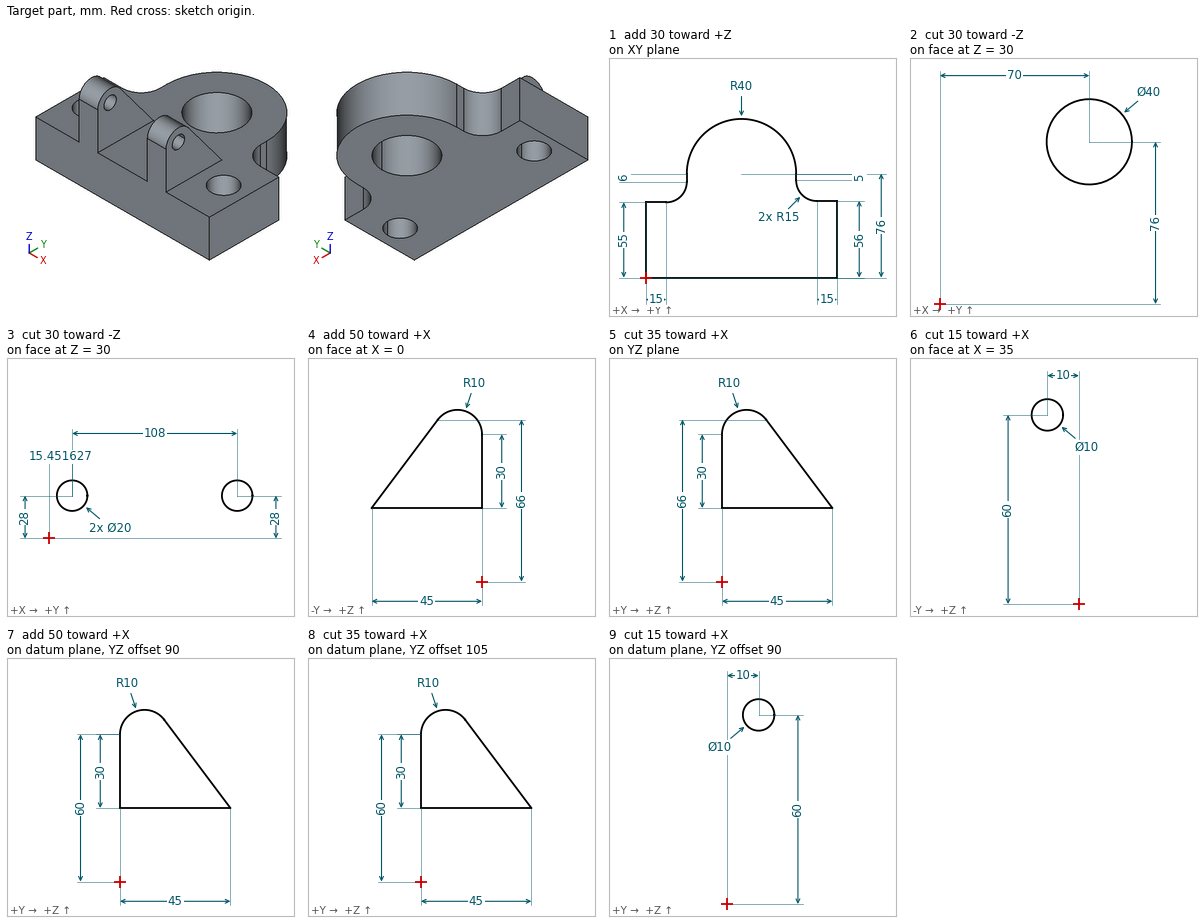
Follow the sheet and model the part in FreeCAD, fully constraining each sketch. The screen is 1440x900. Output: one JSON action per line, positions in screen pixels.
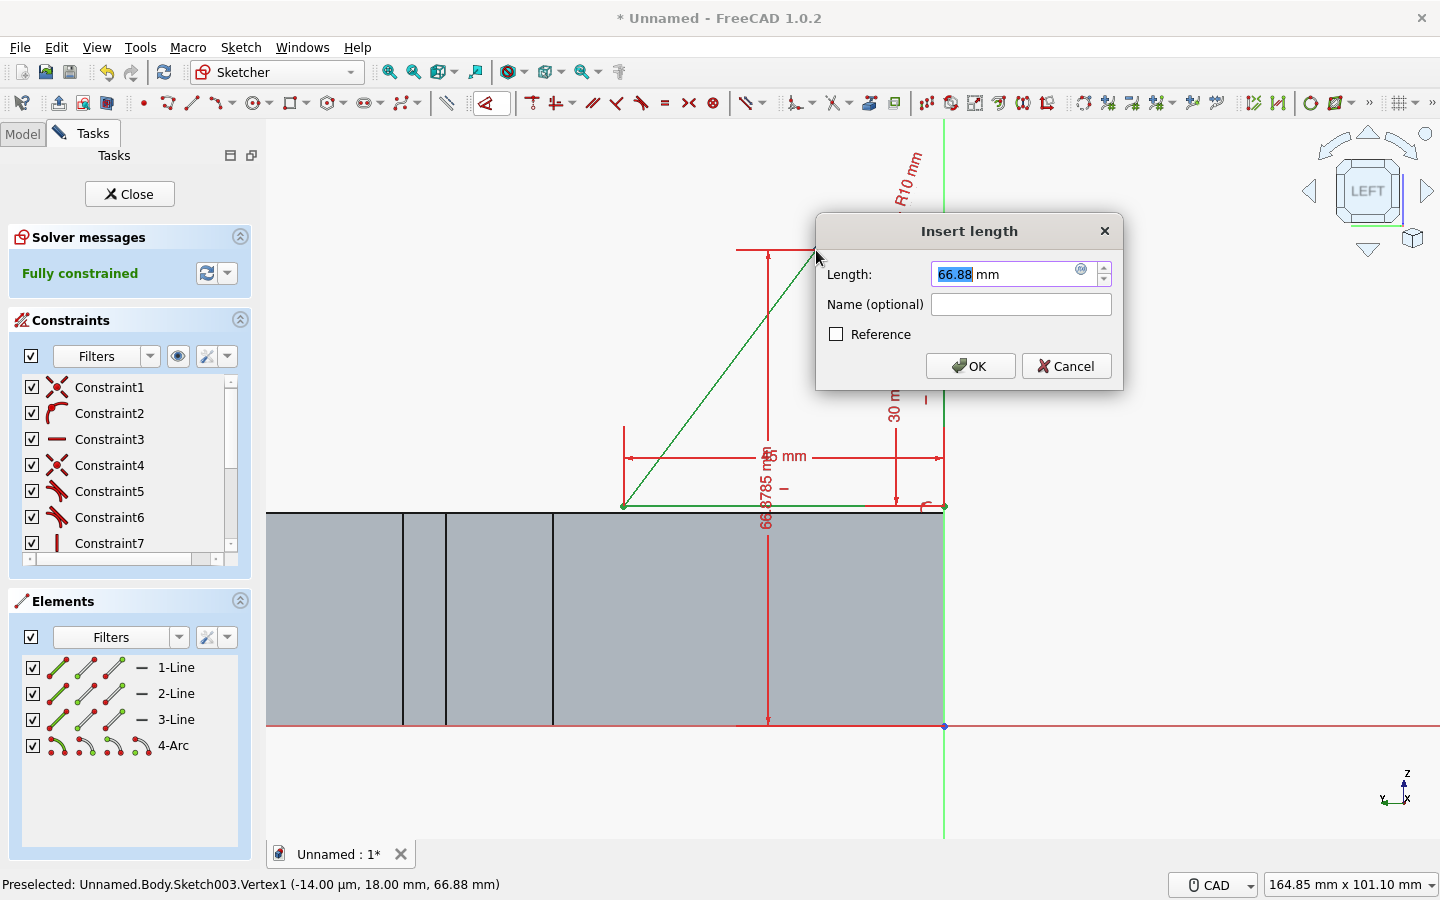
{"action": "type", "text": "66"}
{"action": "key", "text": "Return"}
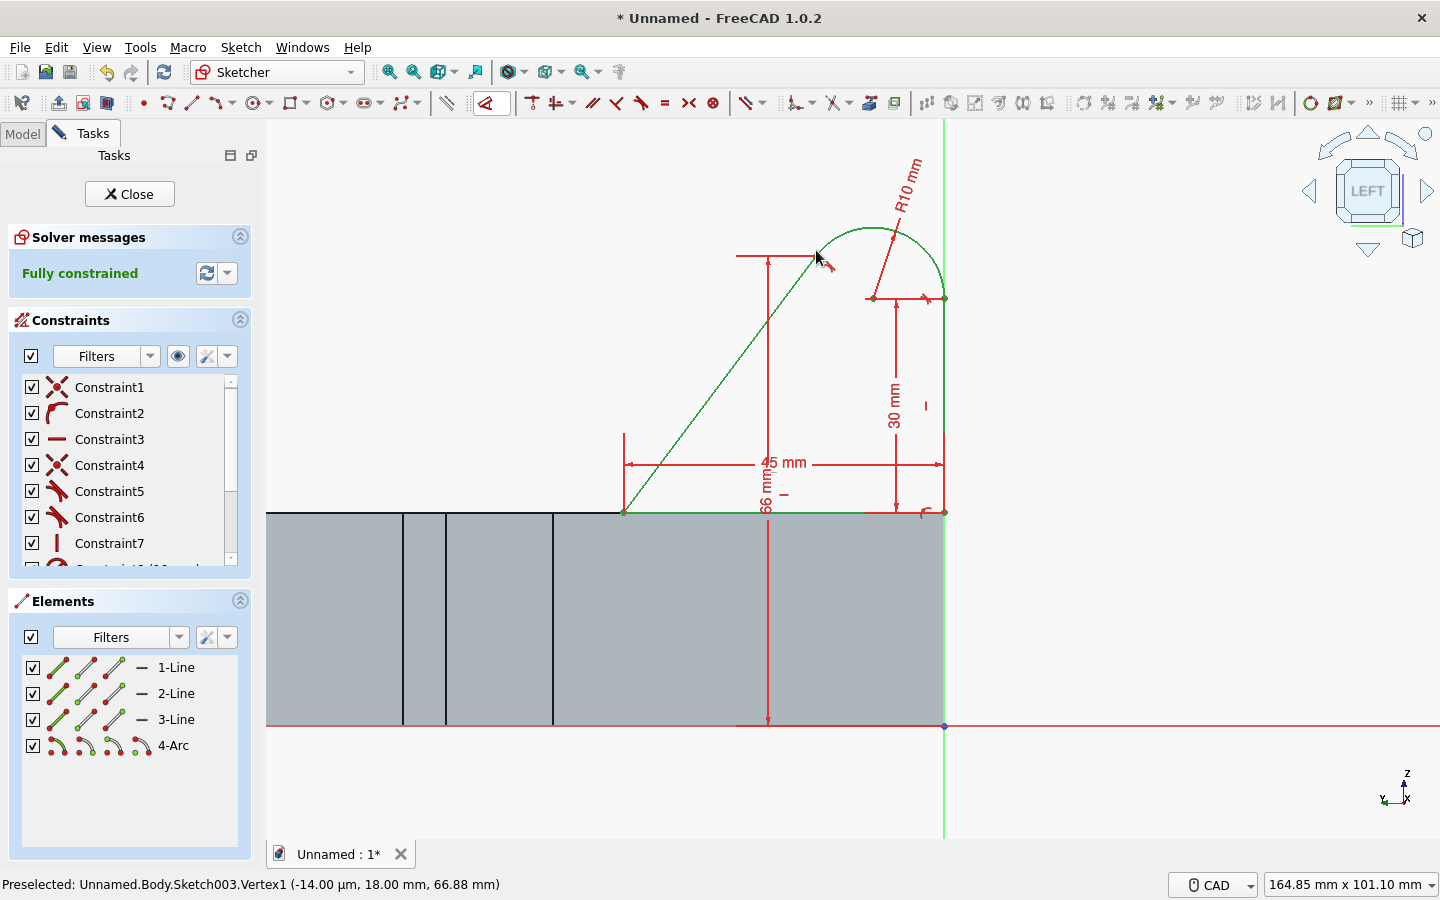
{"action": "left_click", "coordinate": [130, 194]}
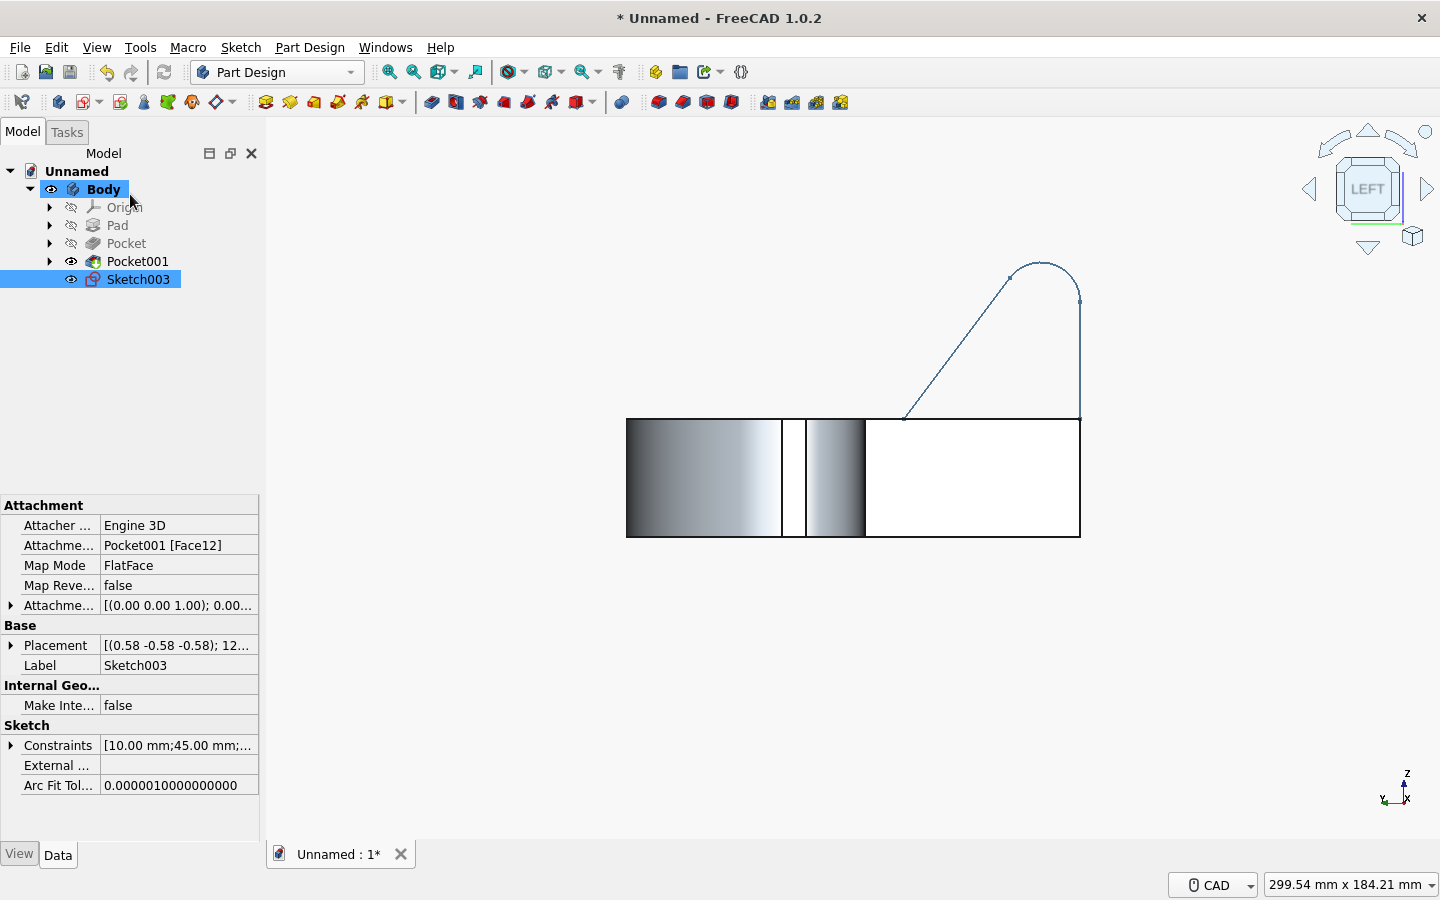
{"action": "left_click", "coordinate": [266, 102]}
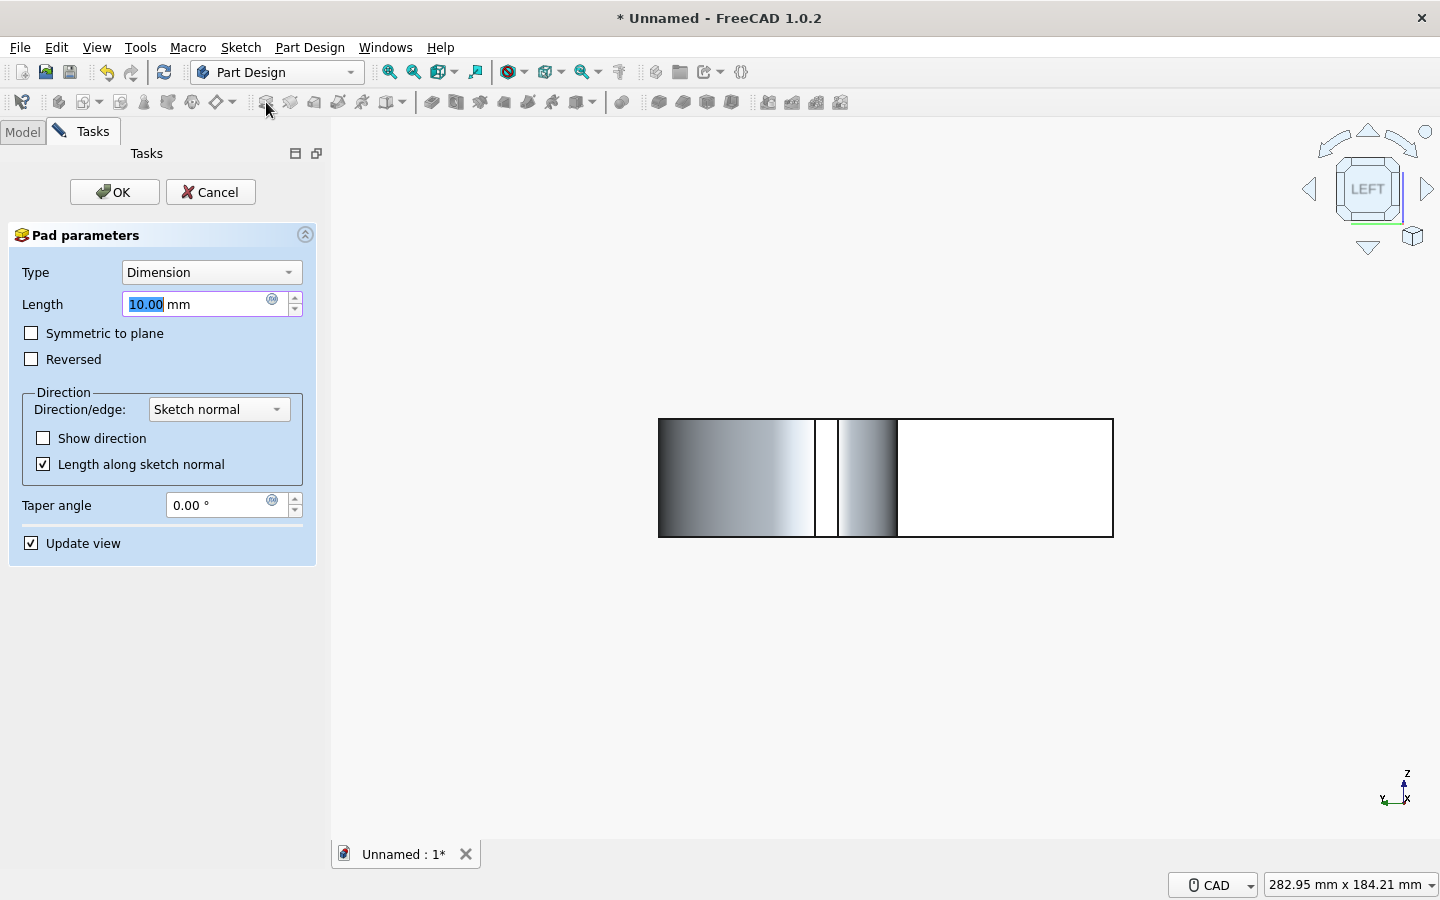
{"action": "type", "text": "50"}
{"action": "key", "text": "Tab"}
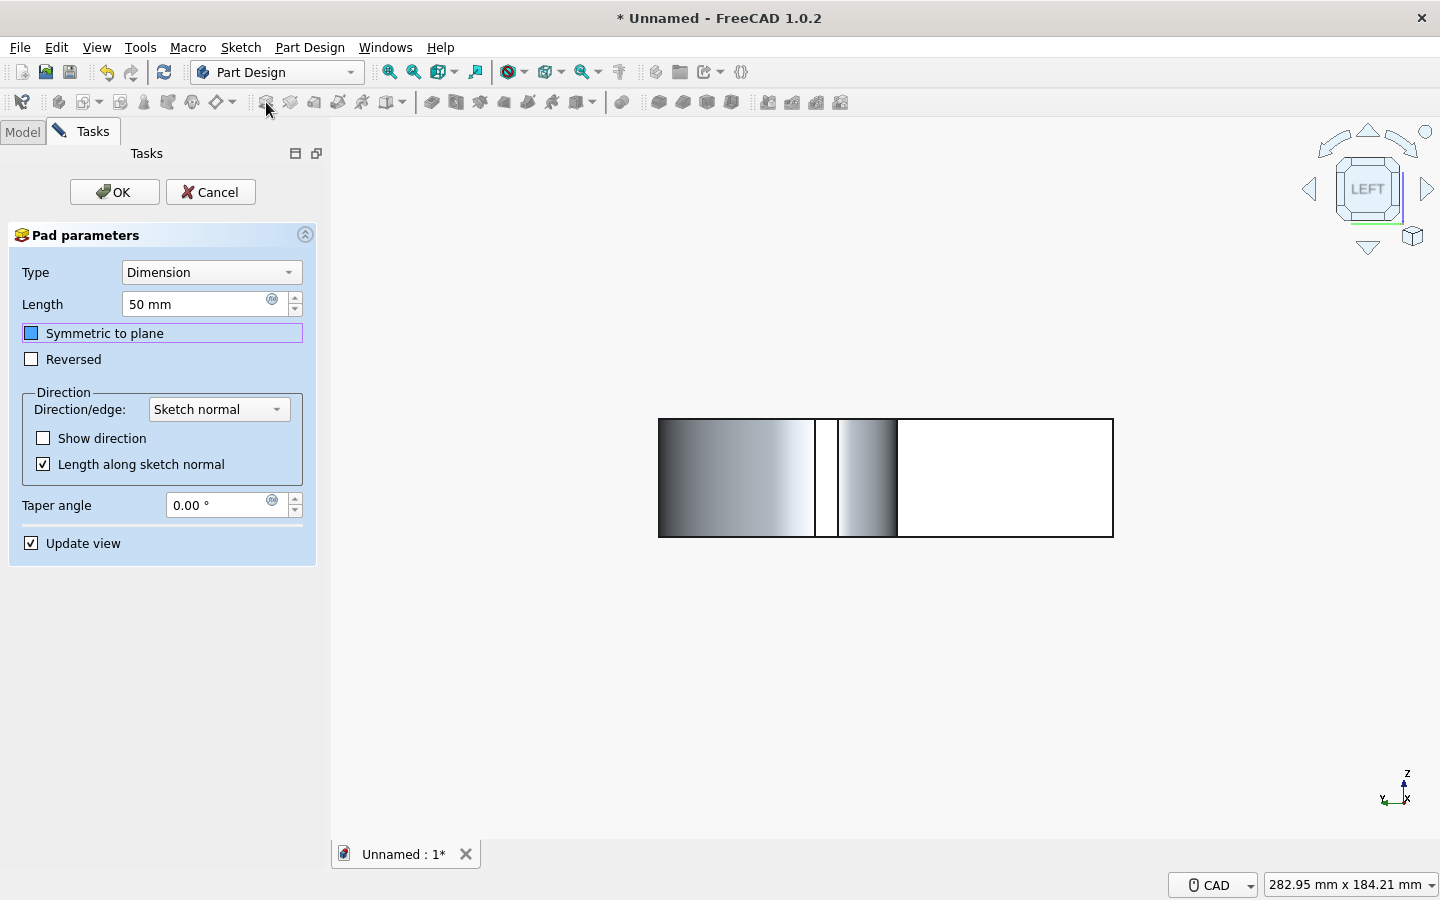
{"action": "left_click", "coordinate": [30, 359]}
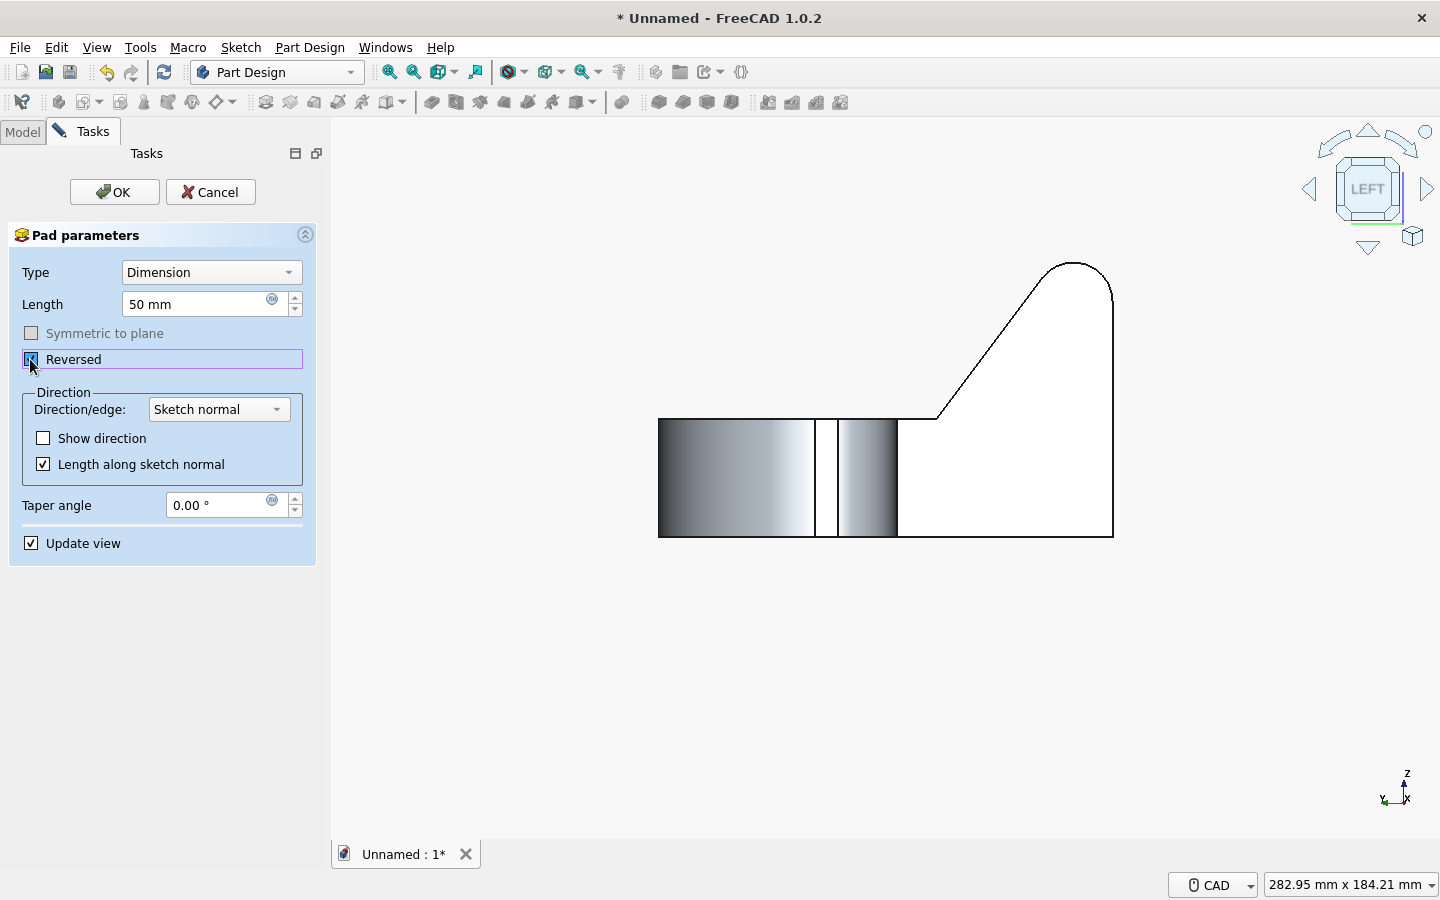
{"action": "left_click", "coordinate": [115, 192]}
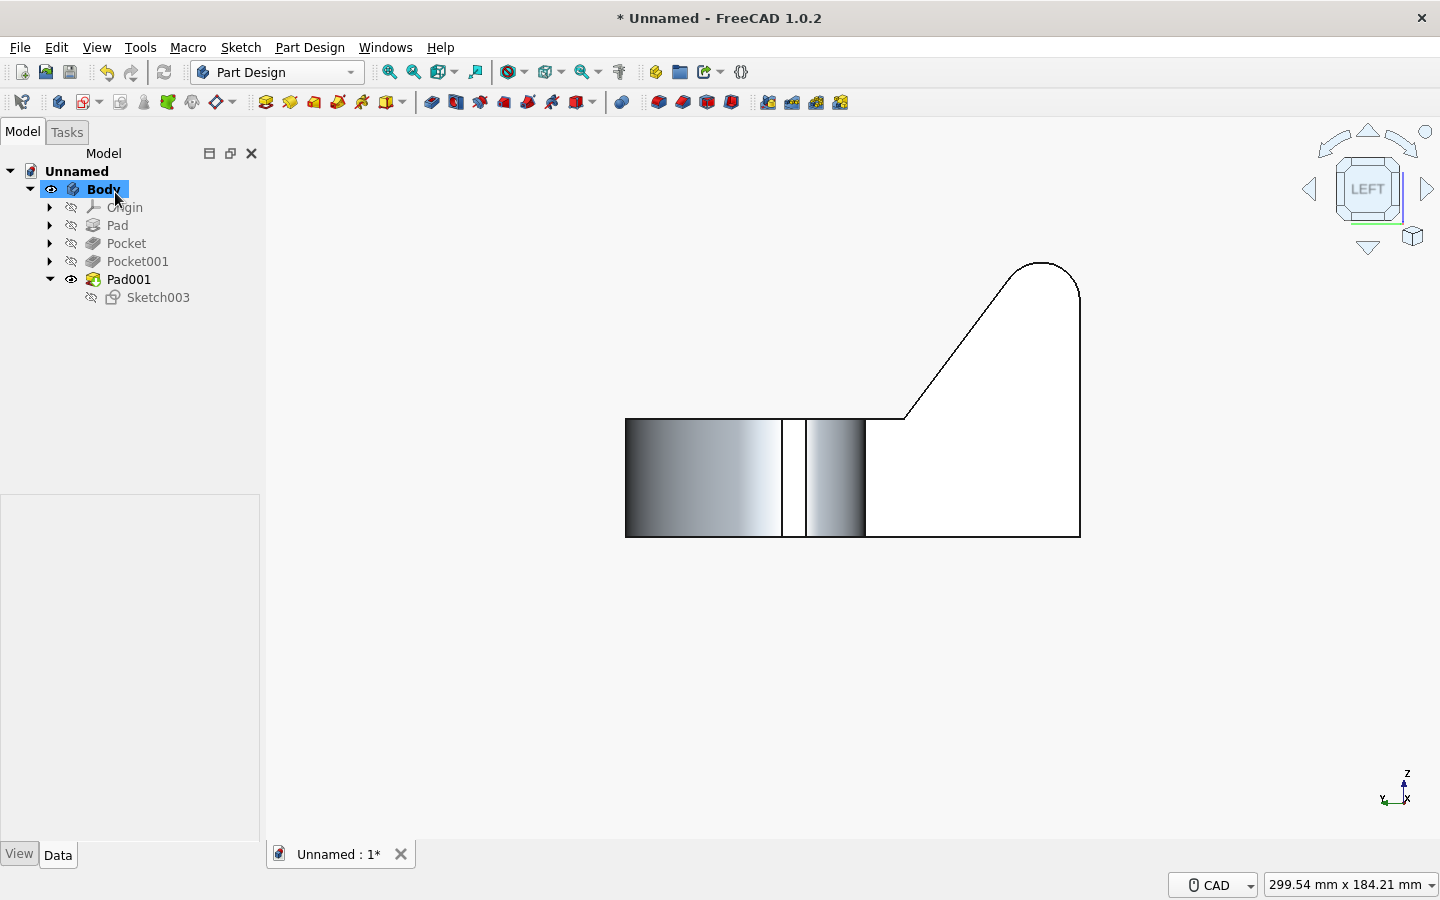
{"action": "key", "text": "v f"}